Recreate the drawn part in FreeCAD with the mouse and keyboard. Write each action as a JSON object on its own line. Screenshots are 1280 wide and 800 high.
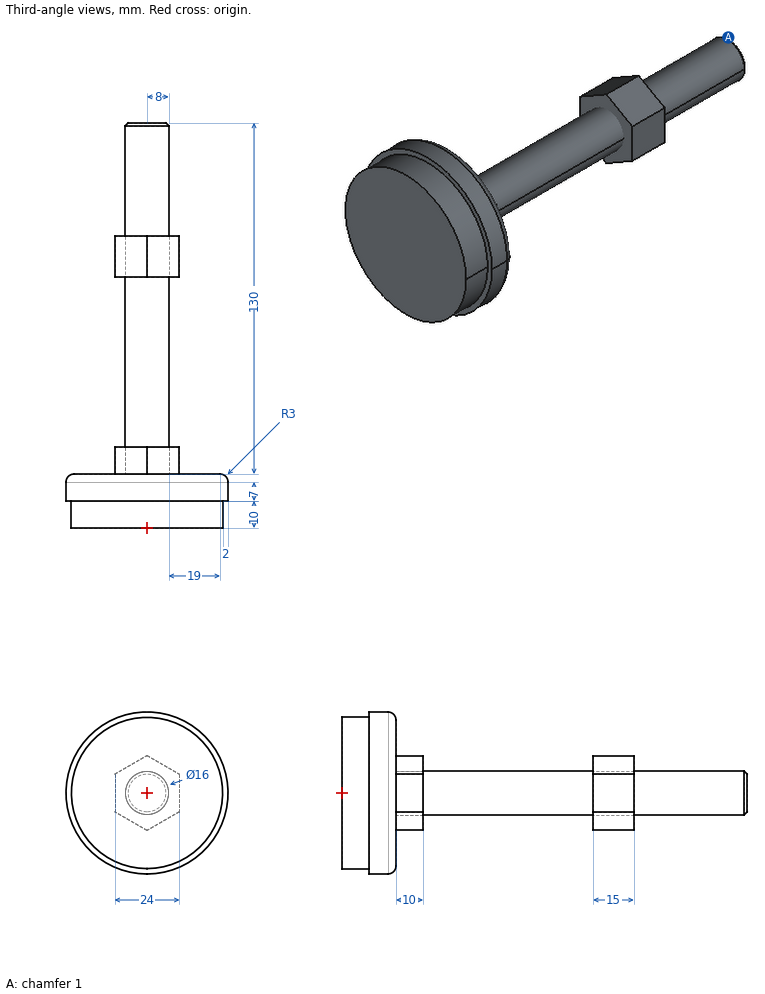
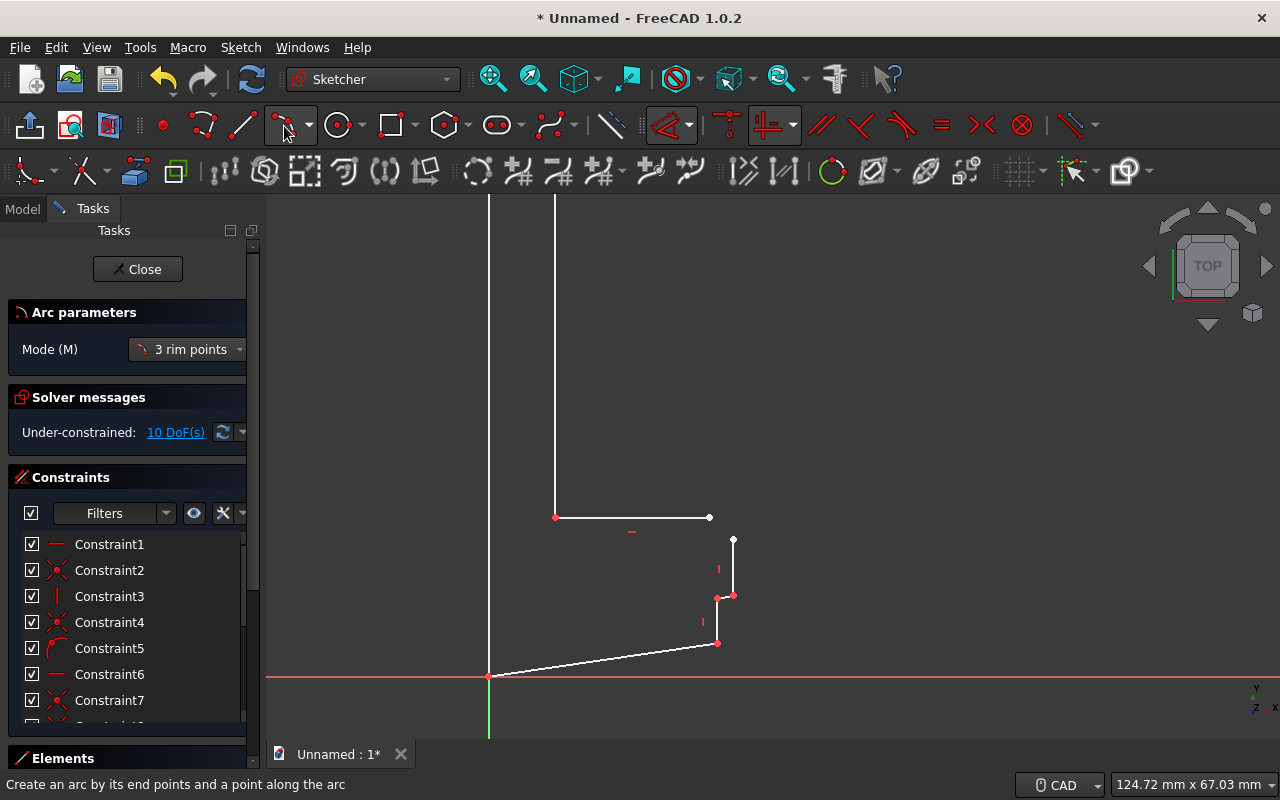
{"action": "left_click", "coordinate": [733, 540]}
{"action": "left_click", "coordinate": [709, 518]}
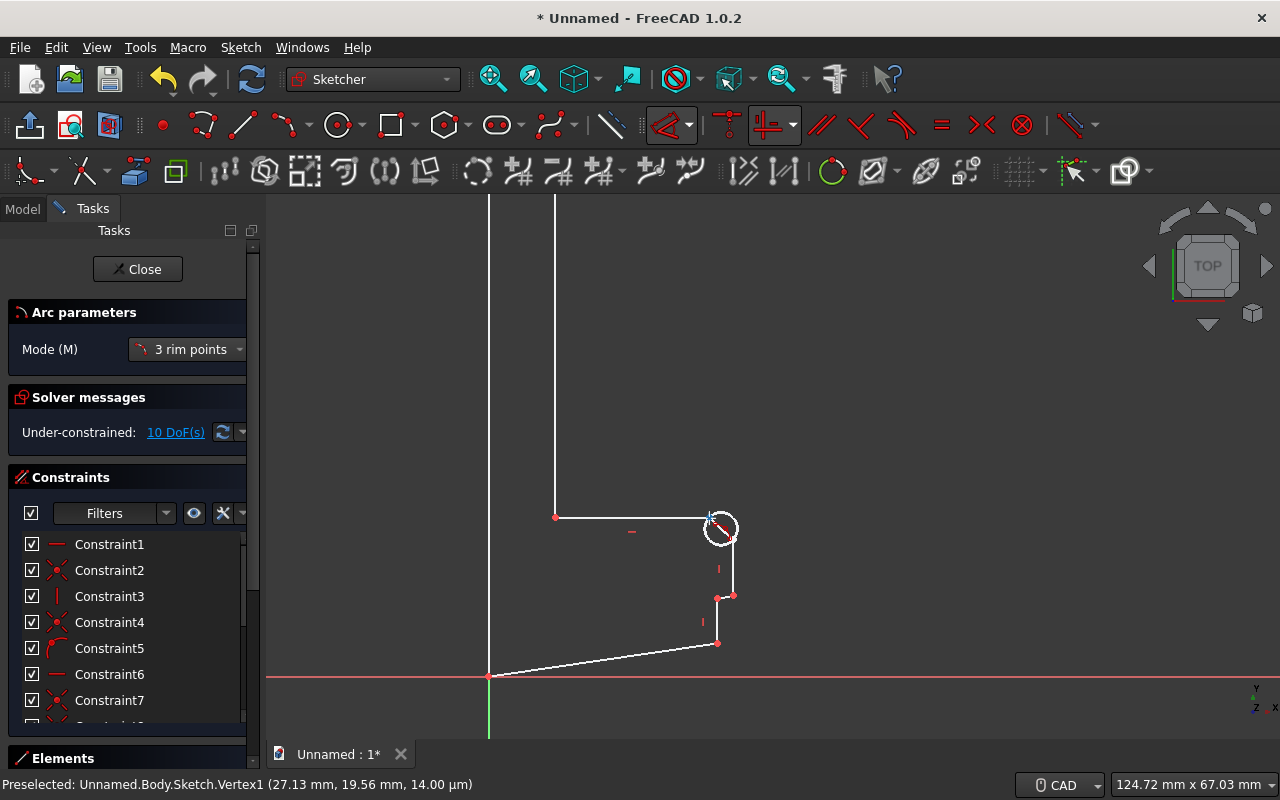
{"action": "scroll", "coordinate": [725, 521], "scroll_direction": "up", "scroll_amount": 4}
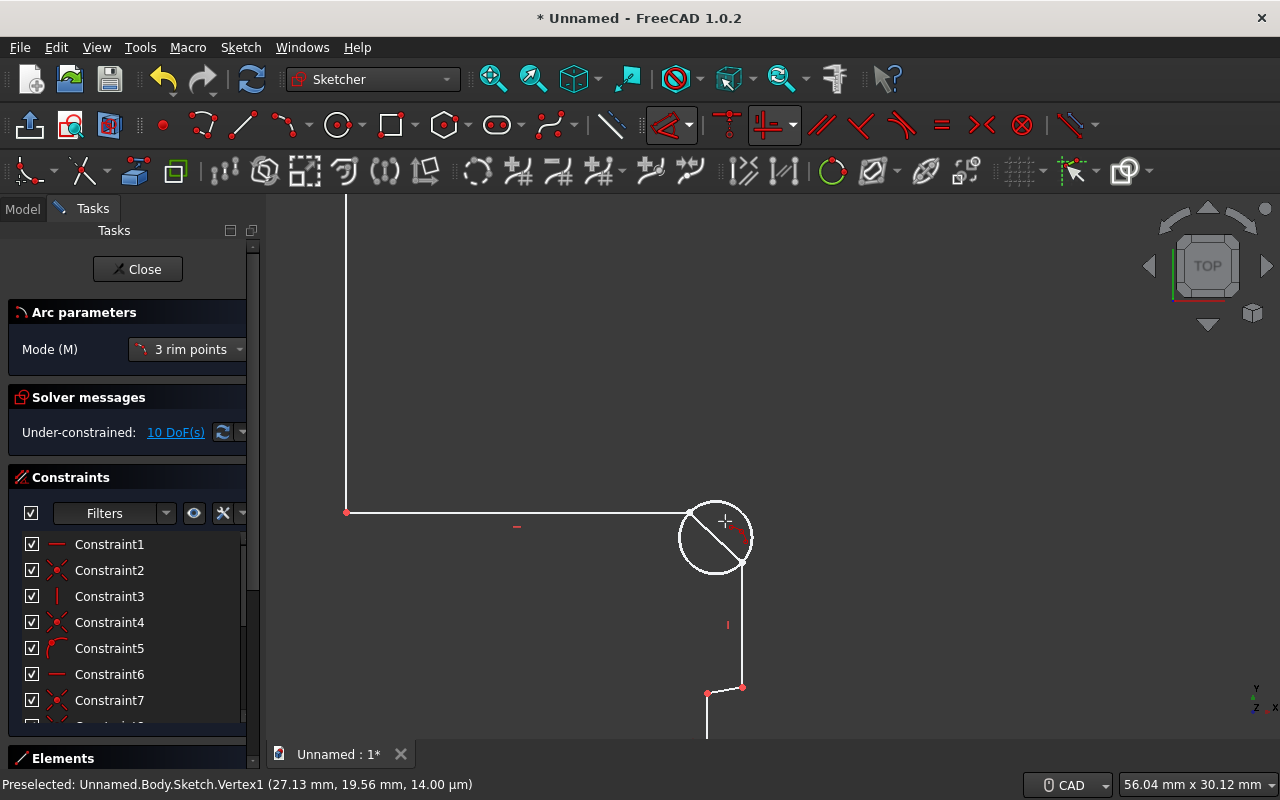
{"action": "left_click", "coordinate": [725, 521]}
{"action": "key", "text": "Escape"}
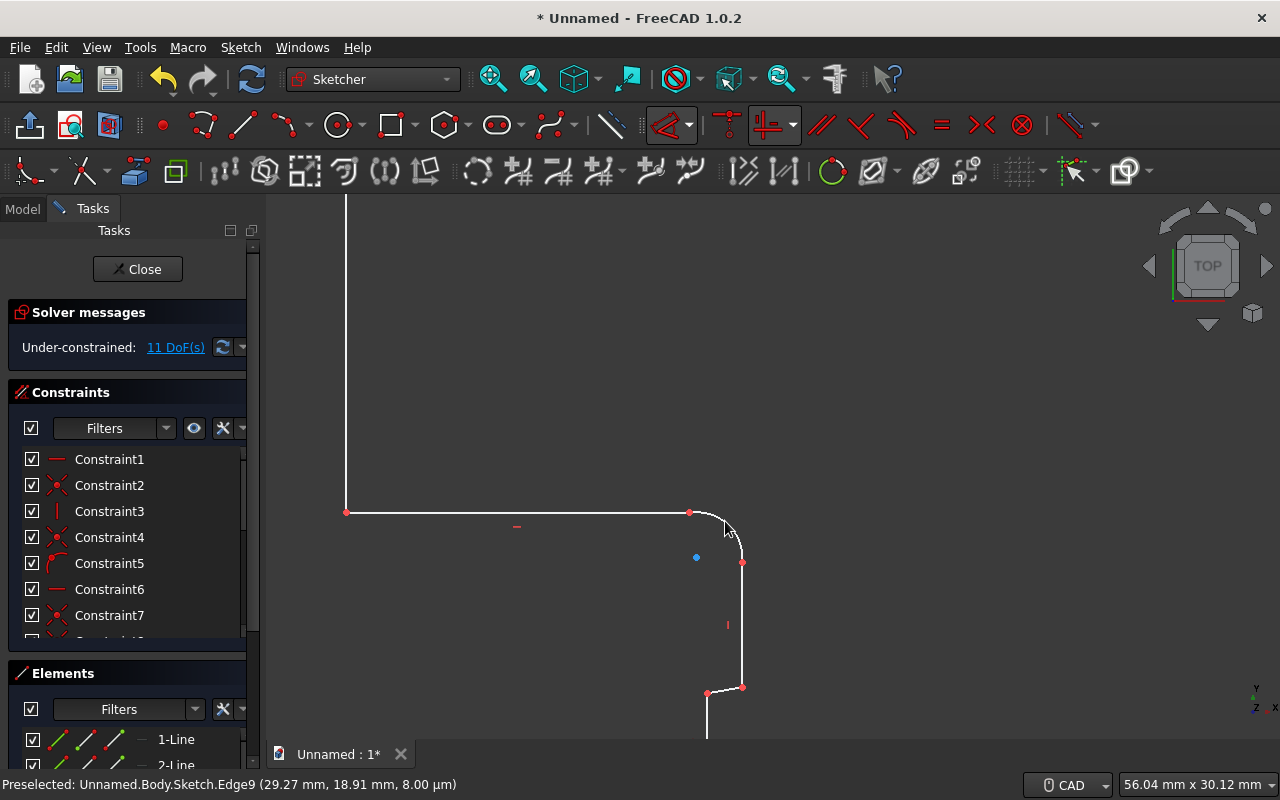
{"action": "scroll", "coordinate": [741, 616], "scroll_direction": "down", "scroll_amount": 10}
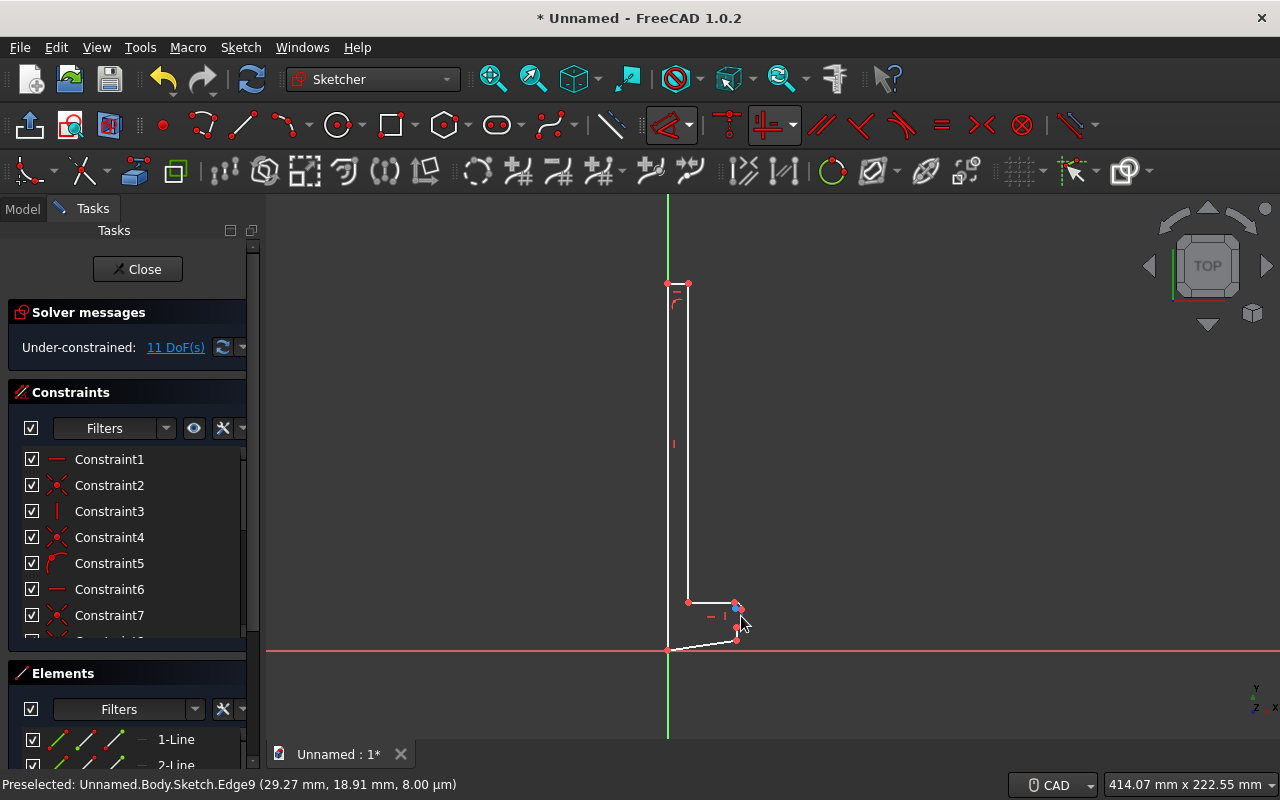
{"action": "left_click", "coordinate": [720, 603]}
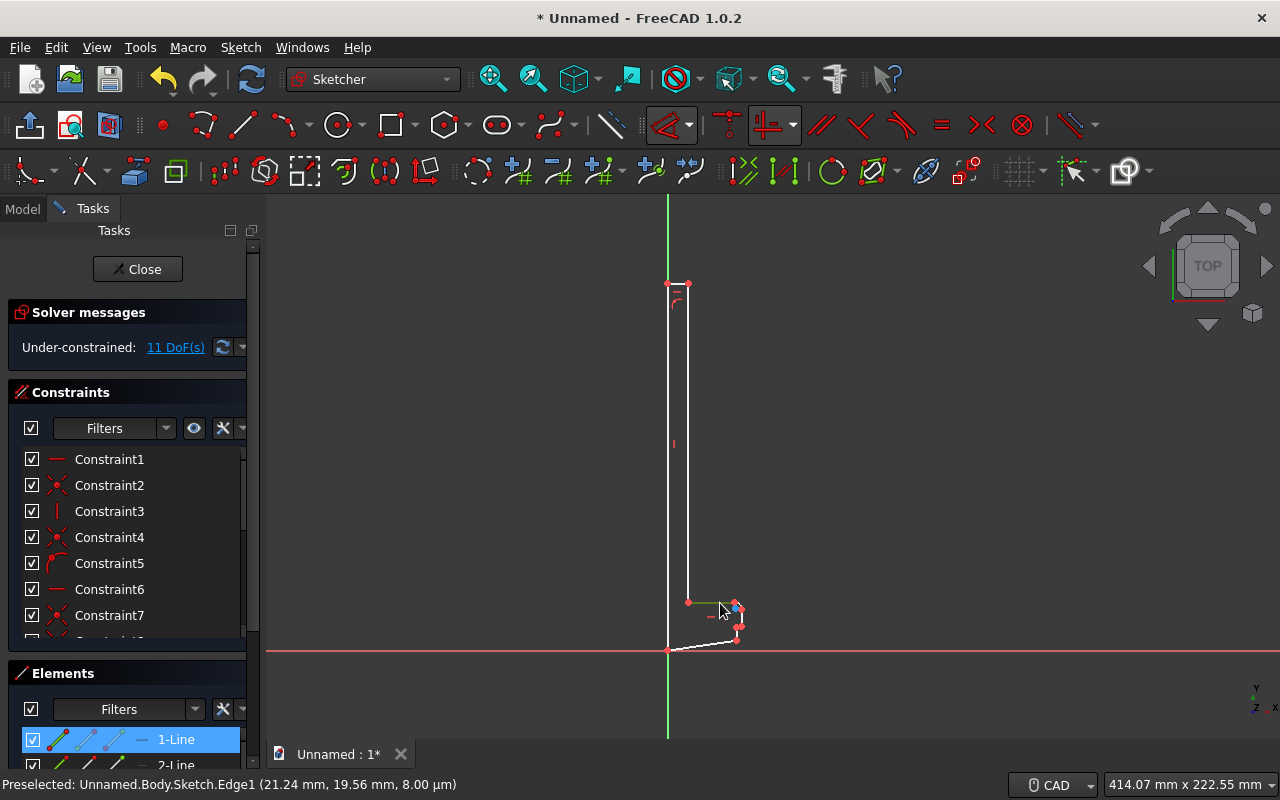
{"action": "scroll", "coordinate": [740, 604], "scroll_direction": "up", "scroll_amount": 5}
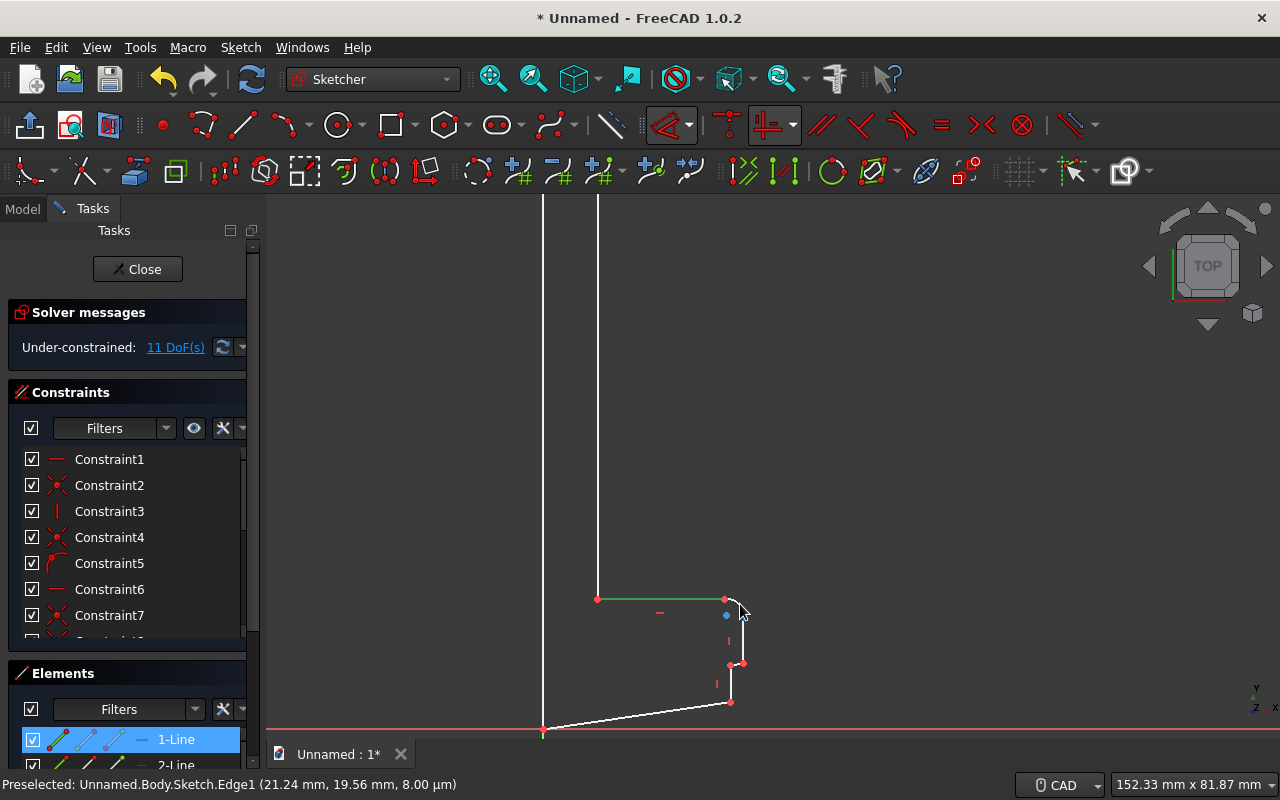
{"action": "left_click", "coordinate": [738, 604]}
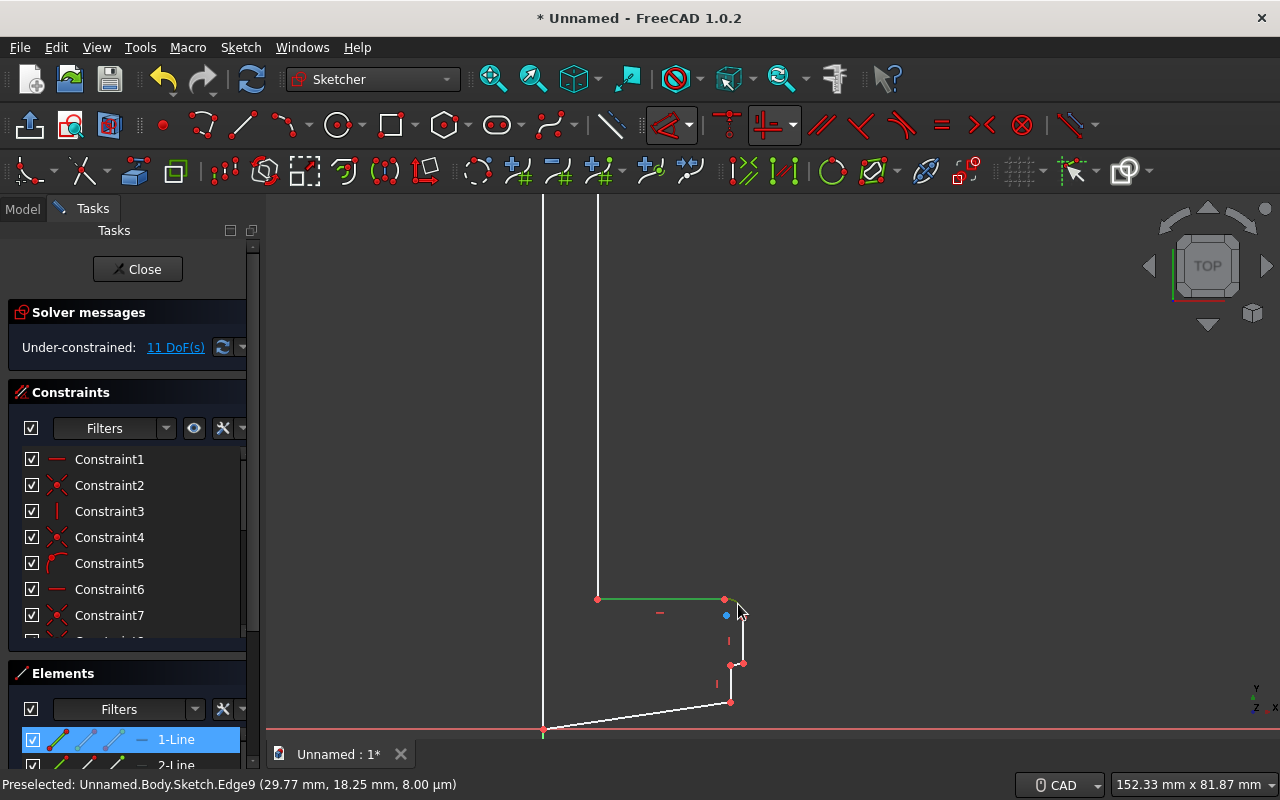
{"action": "left_click", "coordinate": [902, 126]}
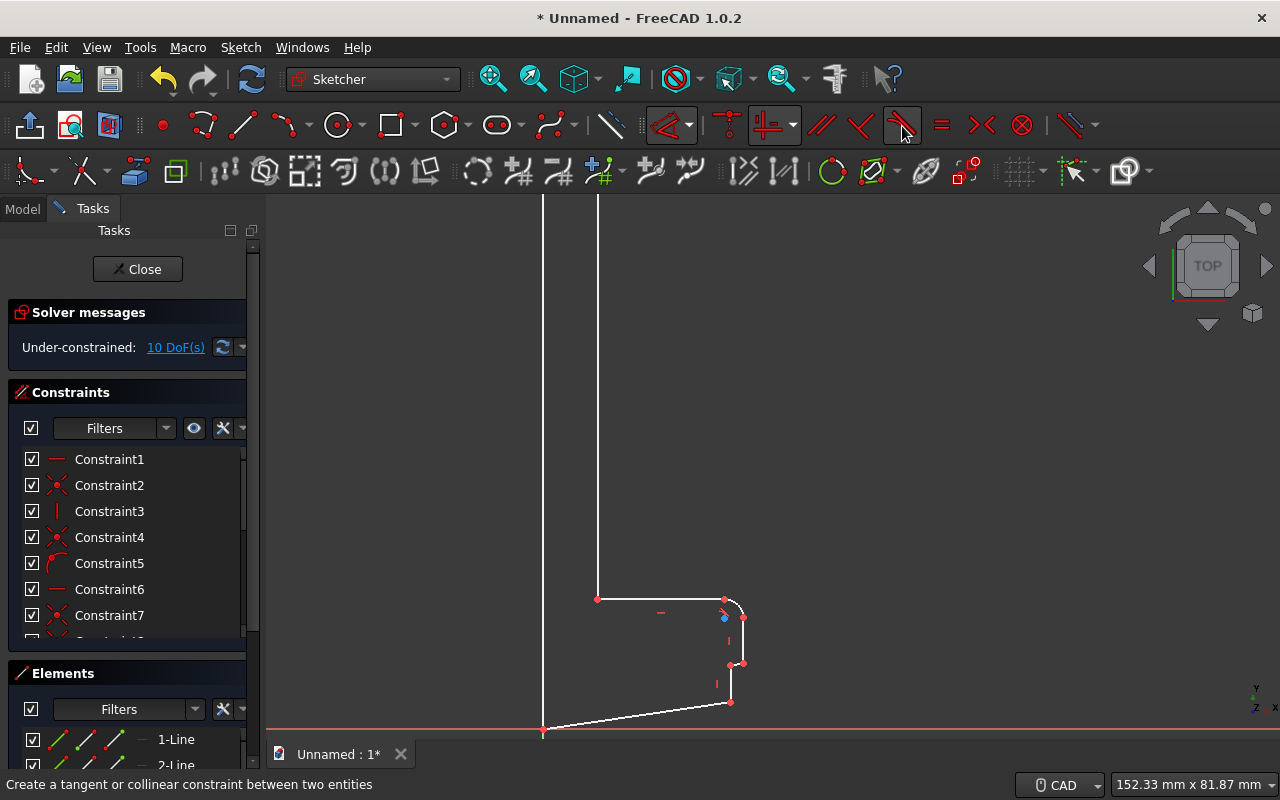
{"action": "left_click", "coordinate": [743, 650]}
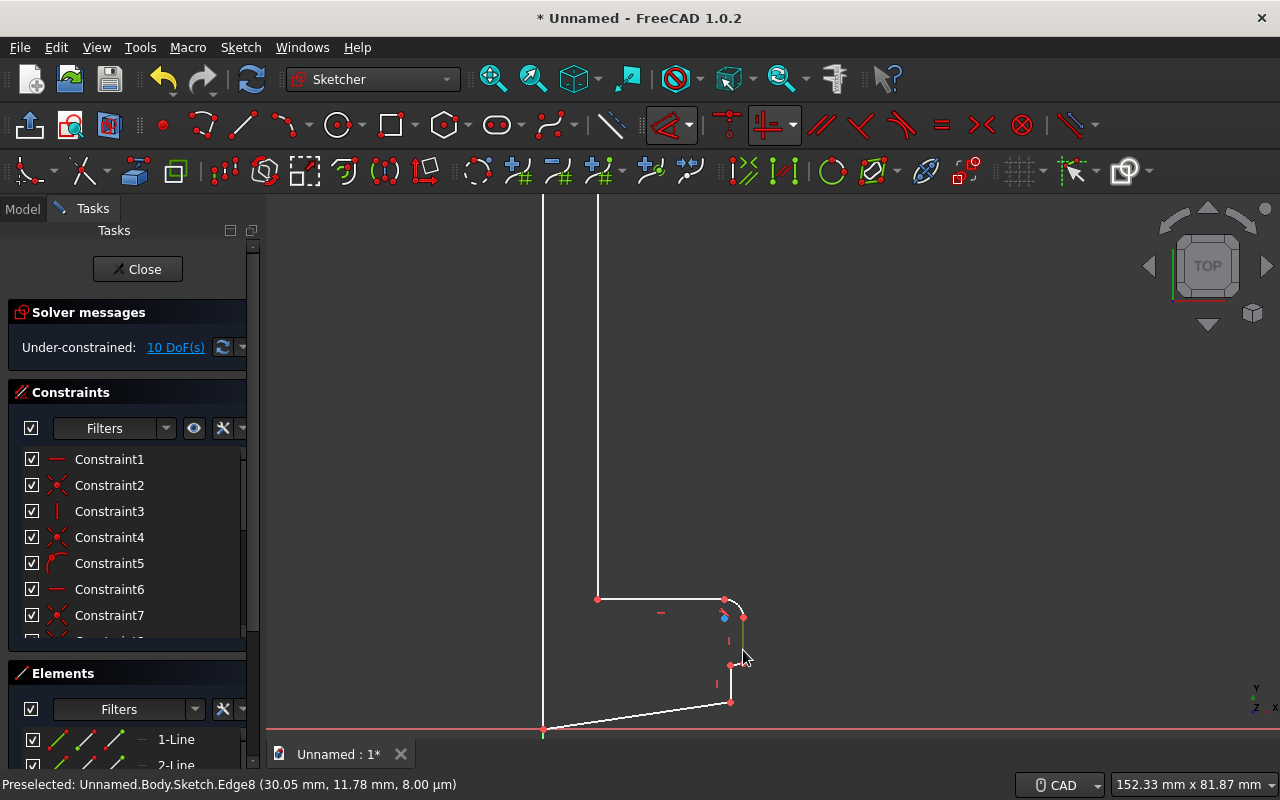
{"action": "left_click", "coordinate": [737, 604]}